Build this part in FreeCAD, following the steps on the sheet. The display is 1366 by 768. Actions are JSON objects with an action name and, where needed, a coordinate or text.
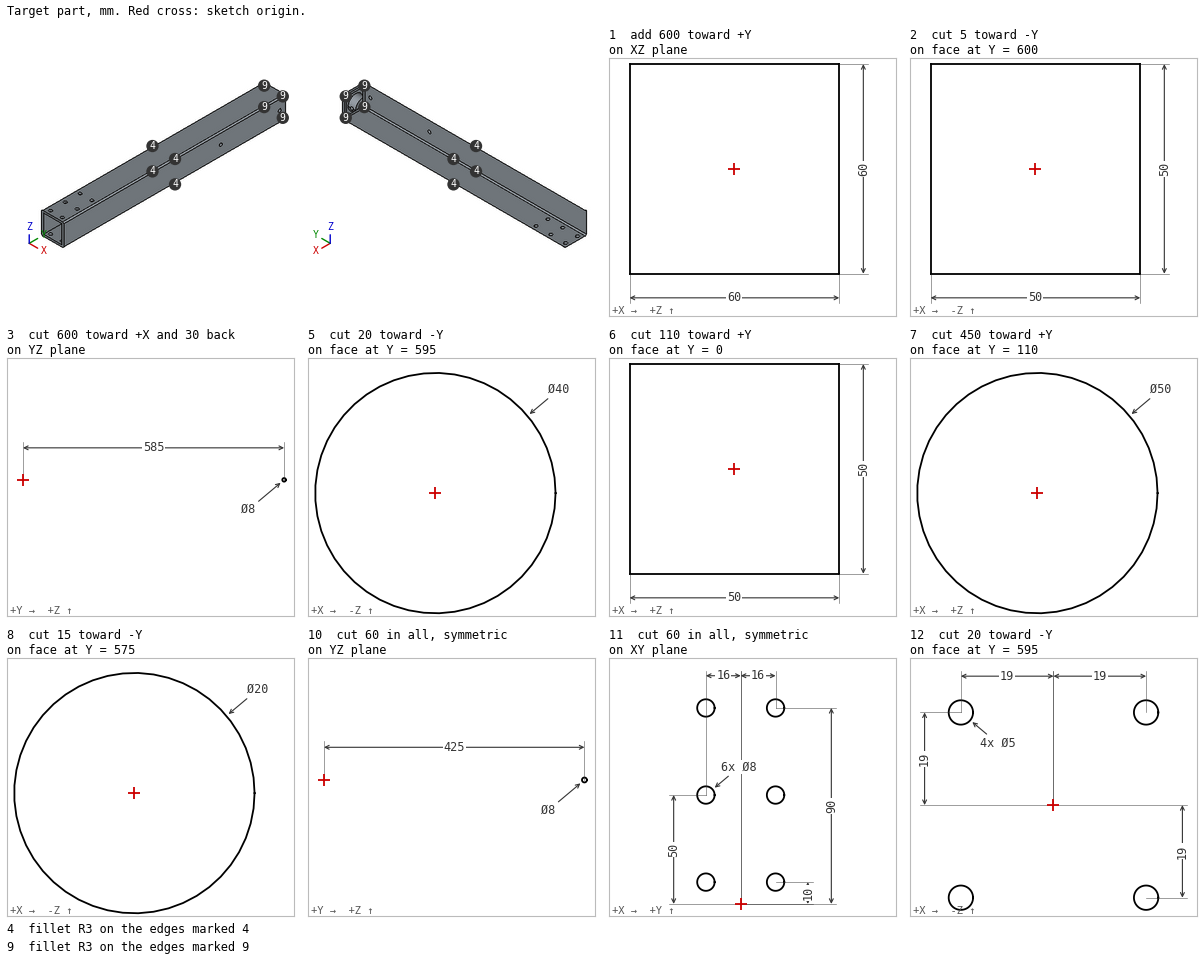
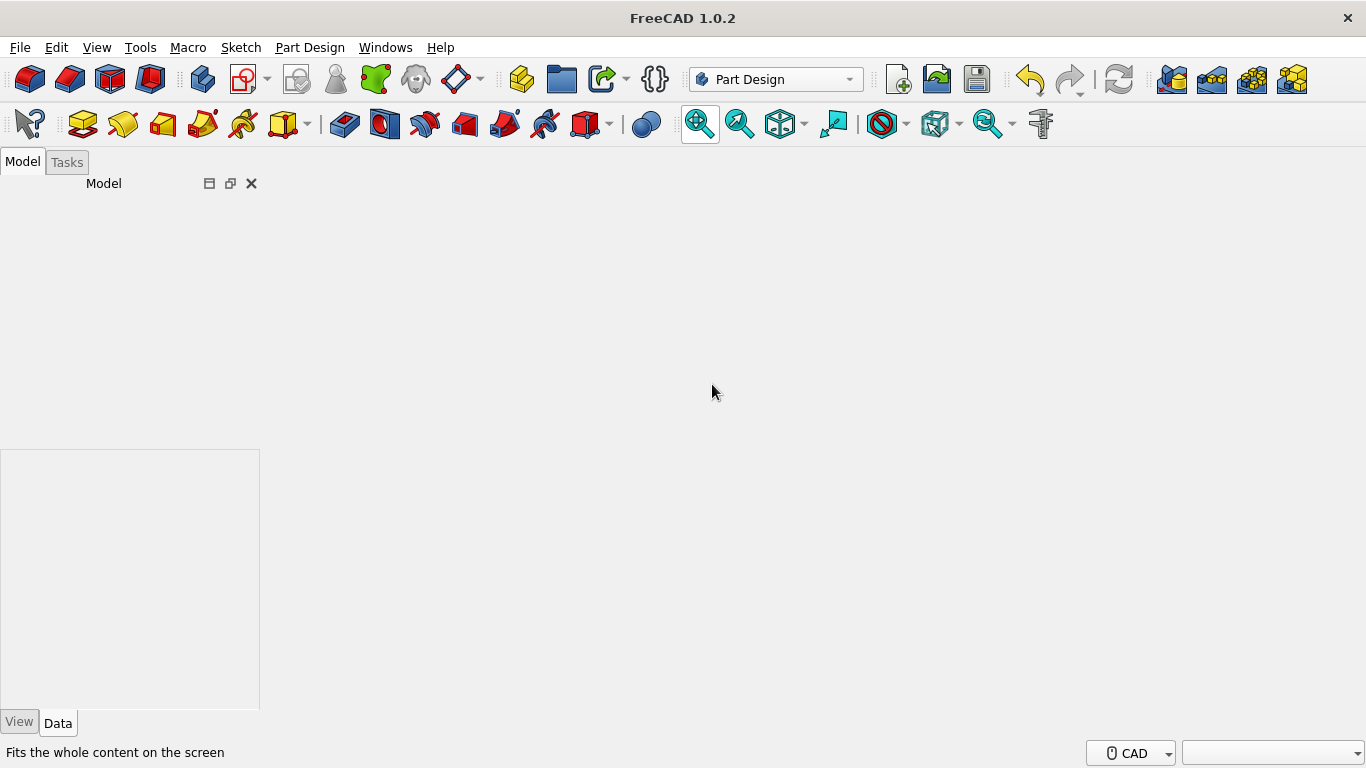
{"action": "left_click", "coordinate": [898, 80]}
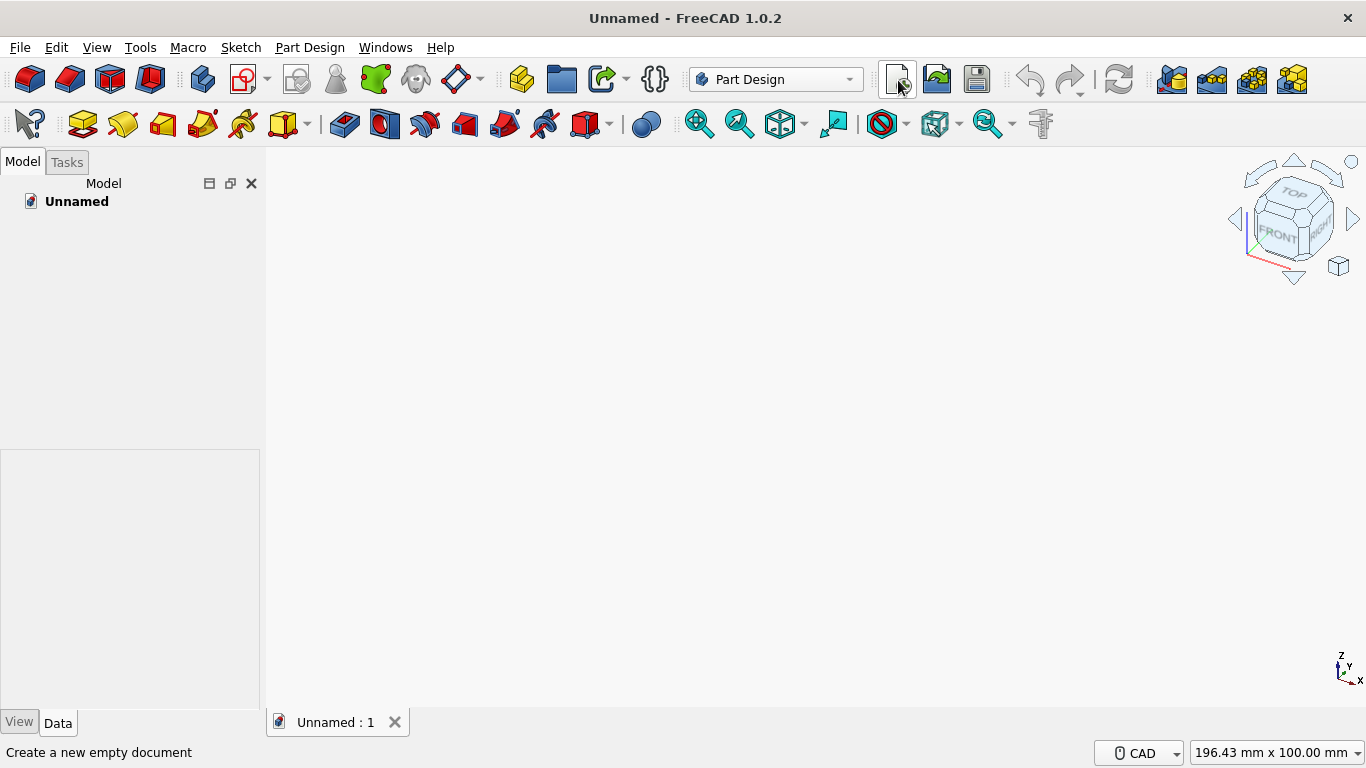
{"action": "left_click", "coordinate": [244, 80]}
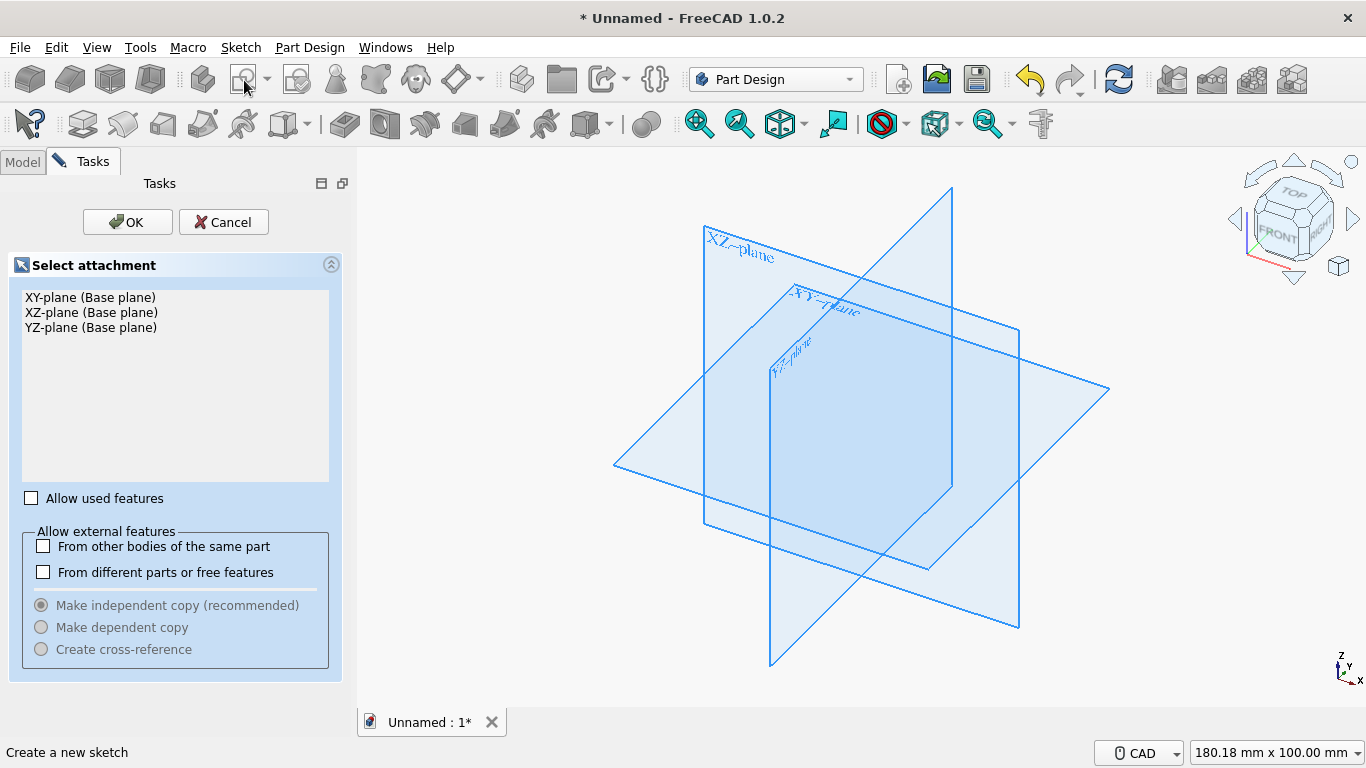
{"action": "left_click", "coordinate": [82, 312]}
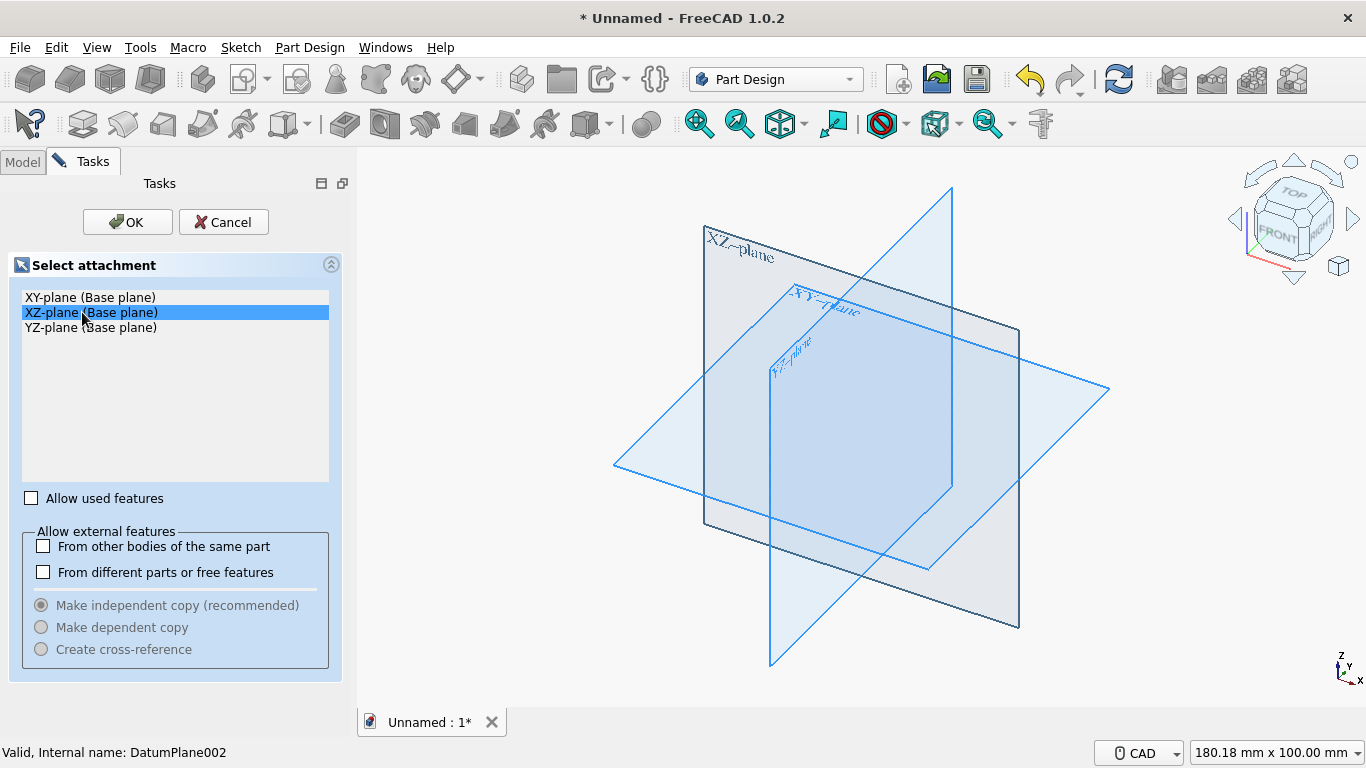
{"action": "left_click", "coordinate": [128, 222]}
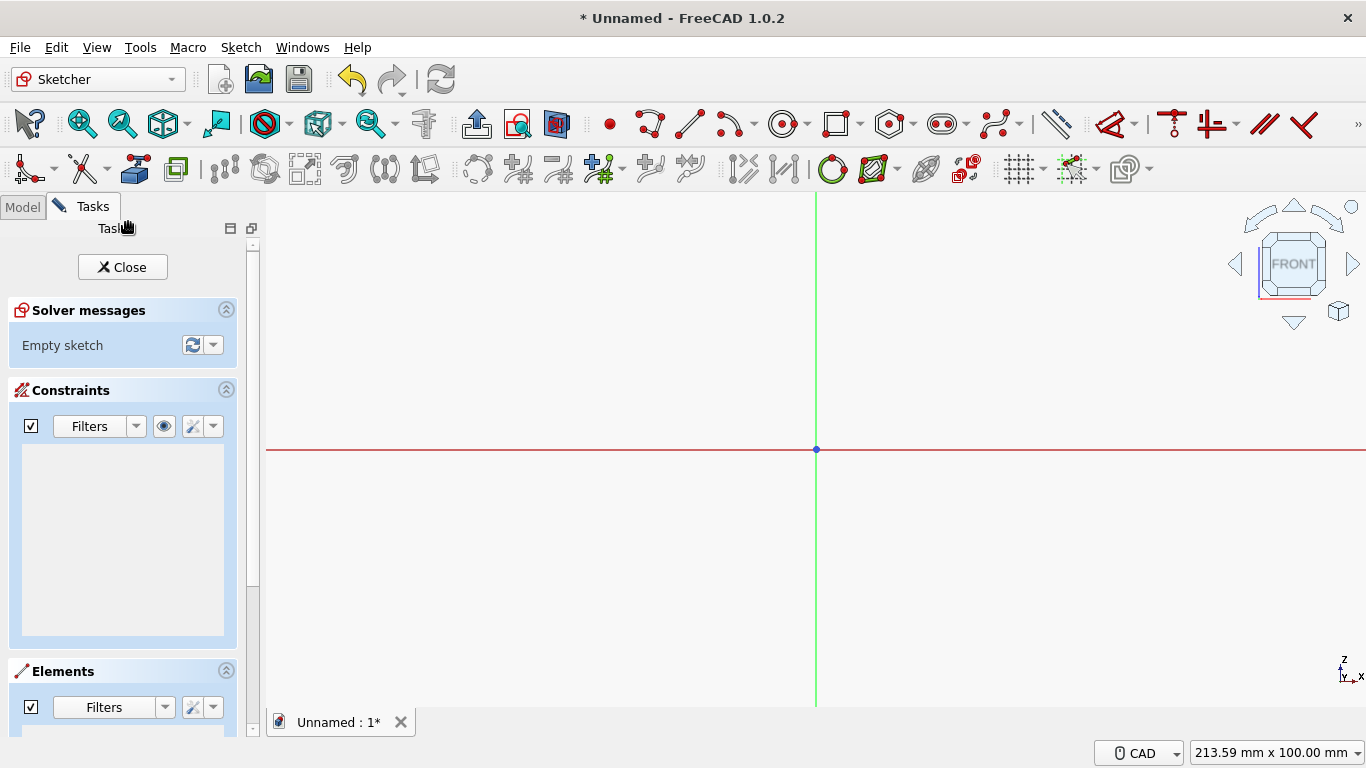
{"action": "left_click", "coordinate": [862, 124]}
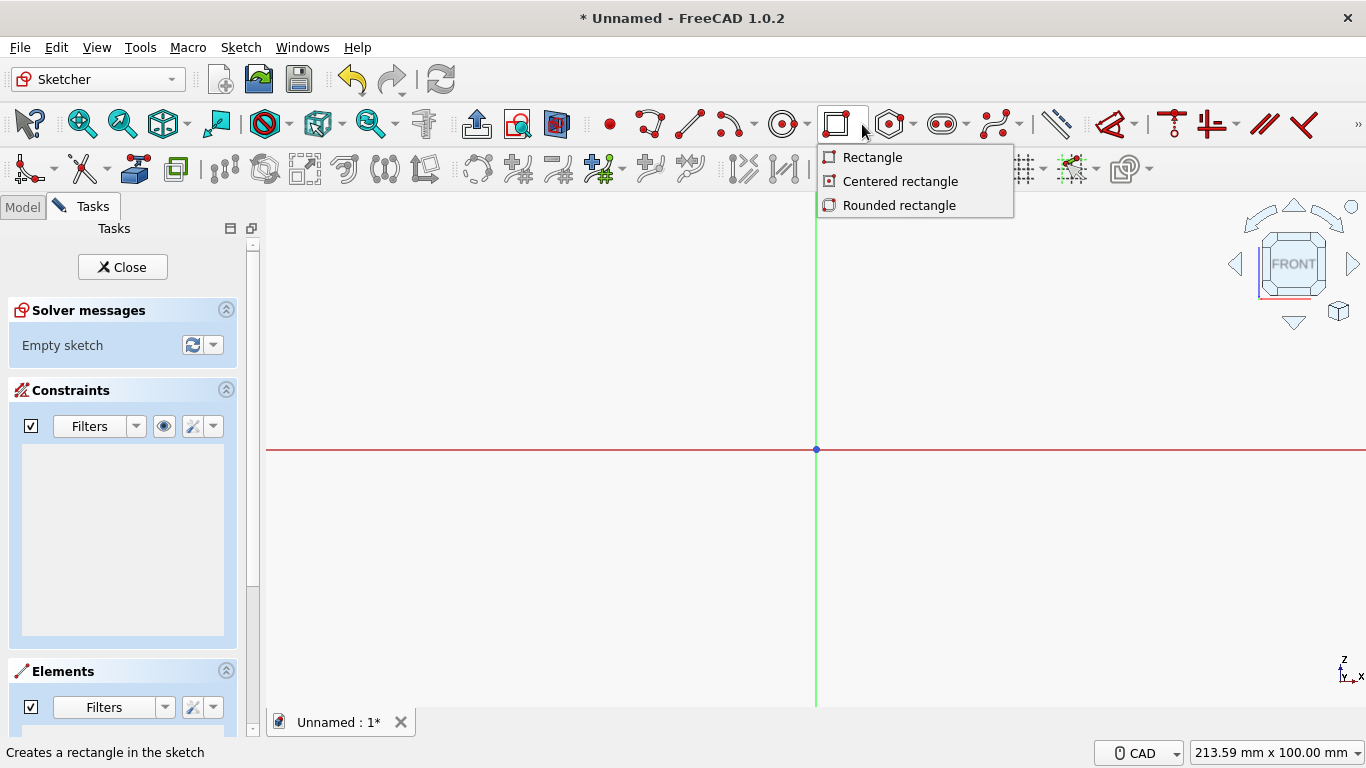
{"action": "left_click", "coordinate": [916, 181]}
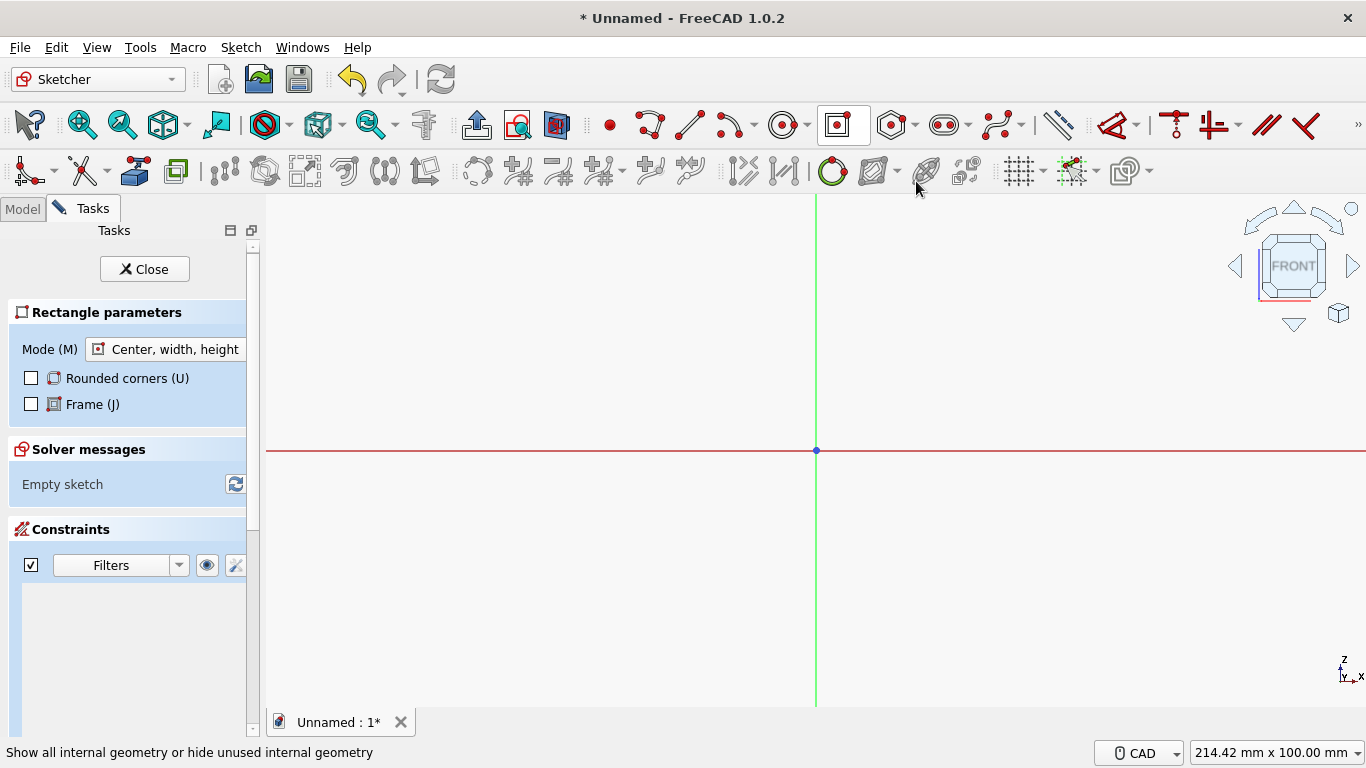
{"action": "left_click", "coordinate": [816, 450]}
{"action": "mouse_move", "coordinate": [970, 297]}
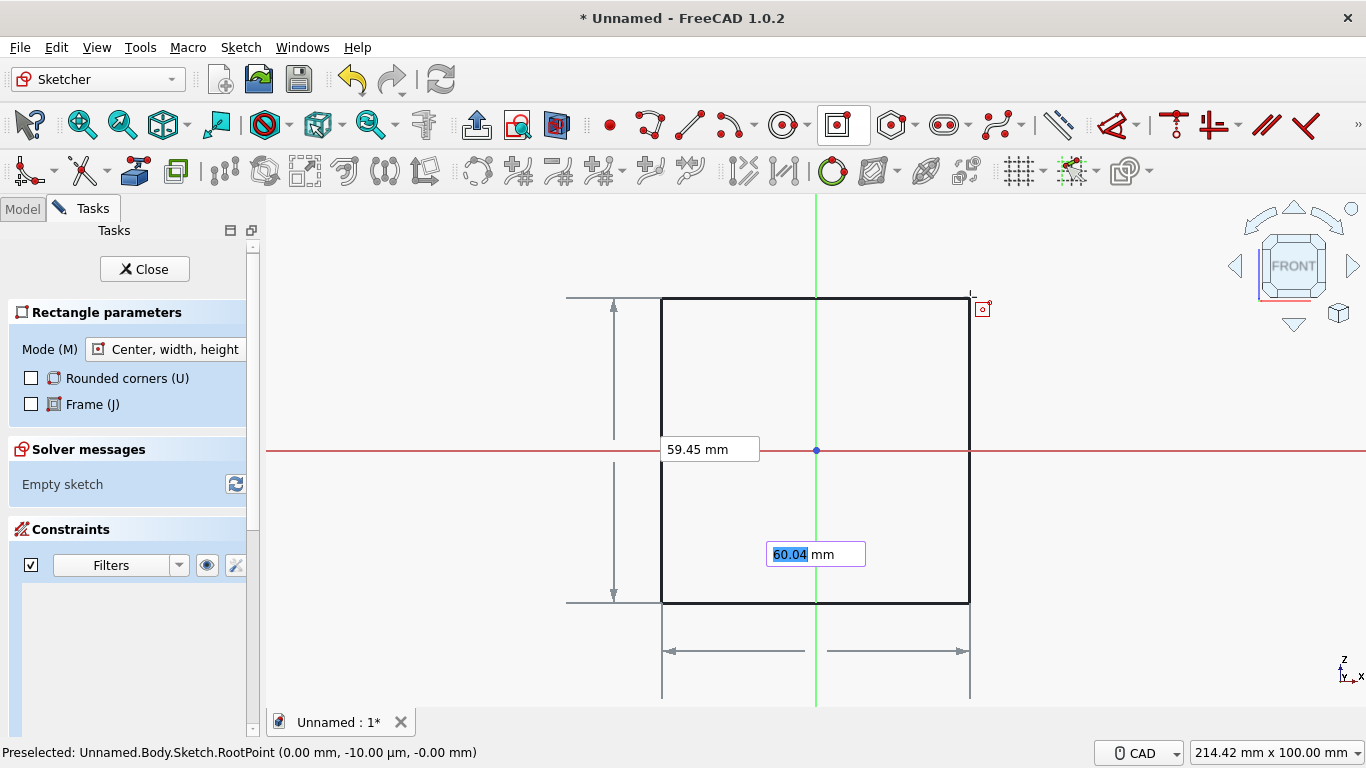
{"action": "type", "text": "60"}
{"action": "key", "text": "Tab"}
{"action": "type", "text": "60"}
{"action": "key", "text": "Return"}
{"action": "key", "text": "Escape"}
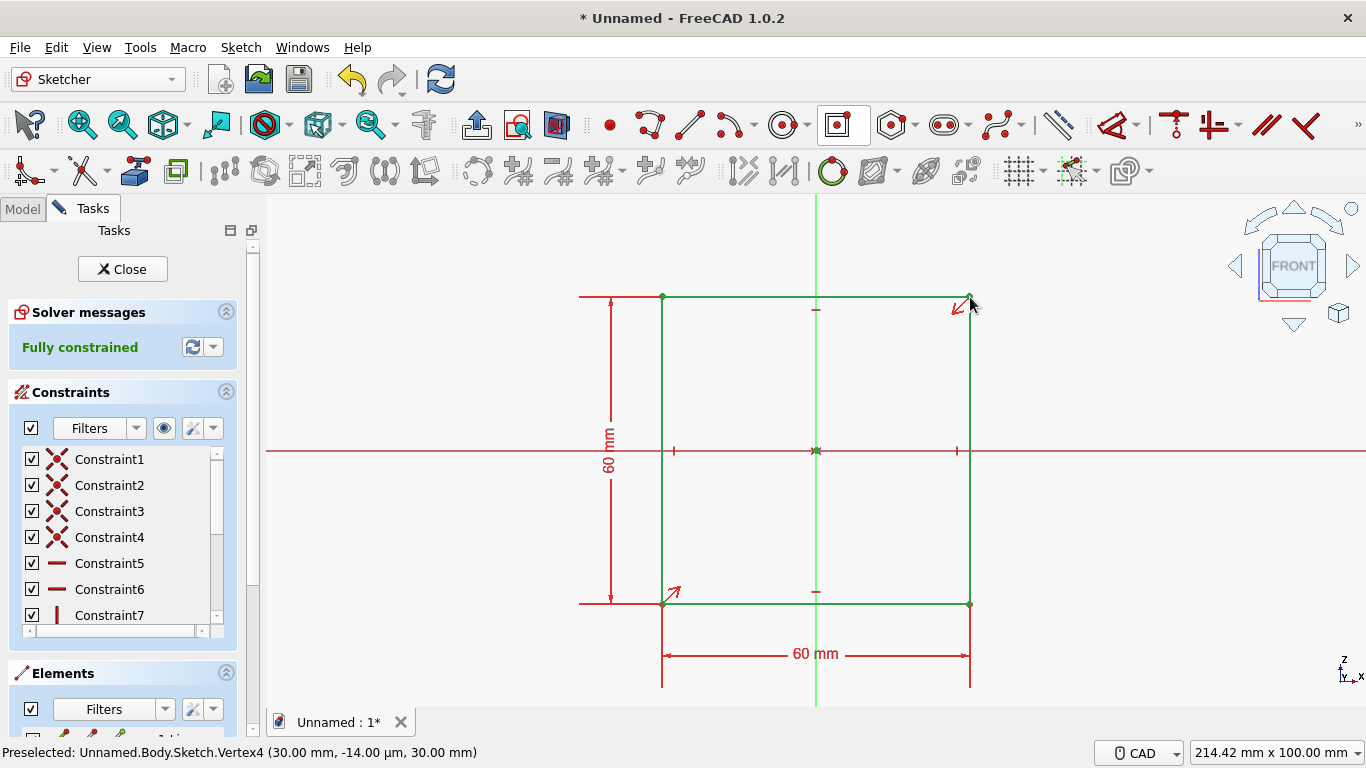
{"action": "left_click", "coordinate": [123, 269]}